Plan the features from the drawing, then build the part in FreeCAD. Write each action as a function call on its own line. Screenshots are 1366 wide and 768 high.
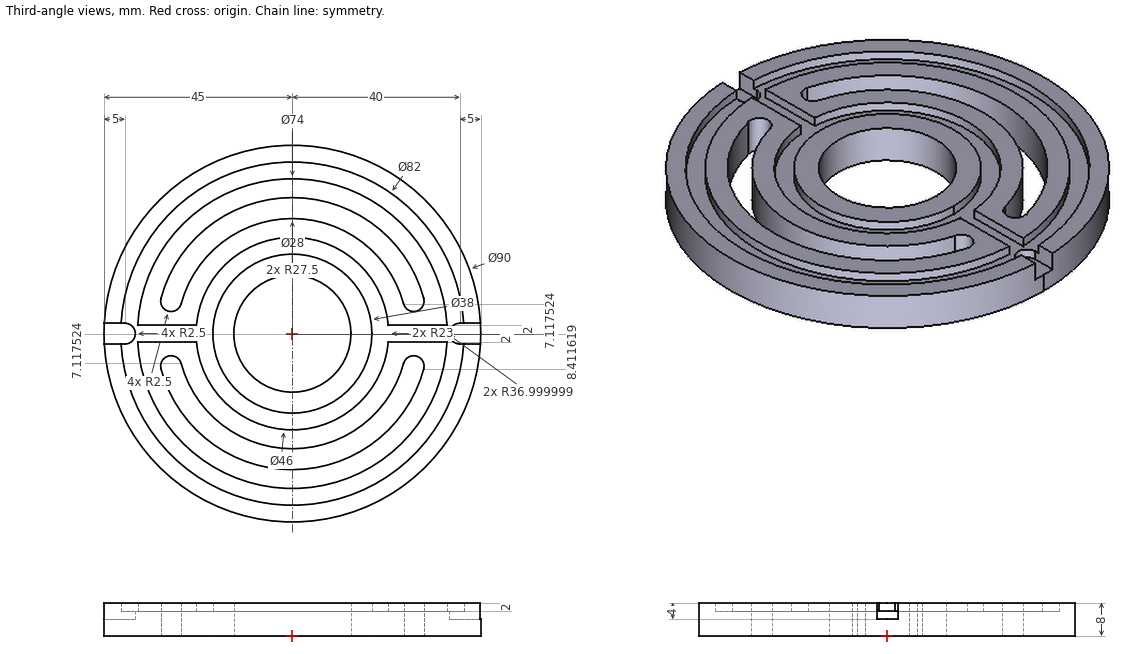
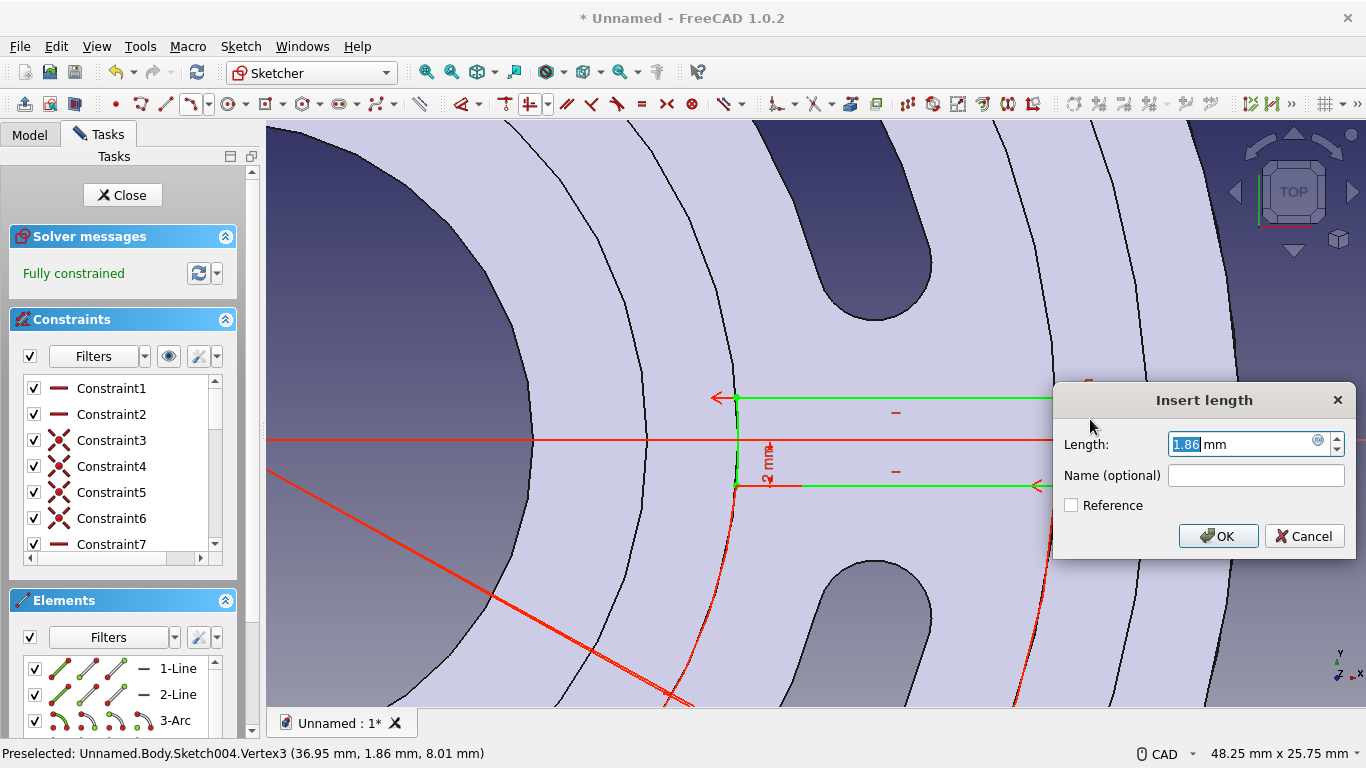
text(2)
key(Return)
key(Escape)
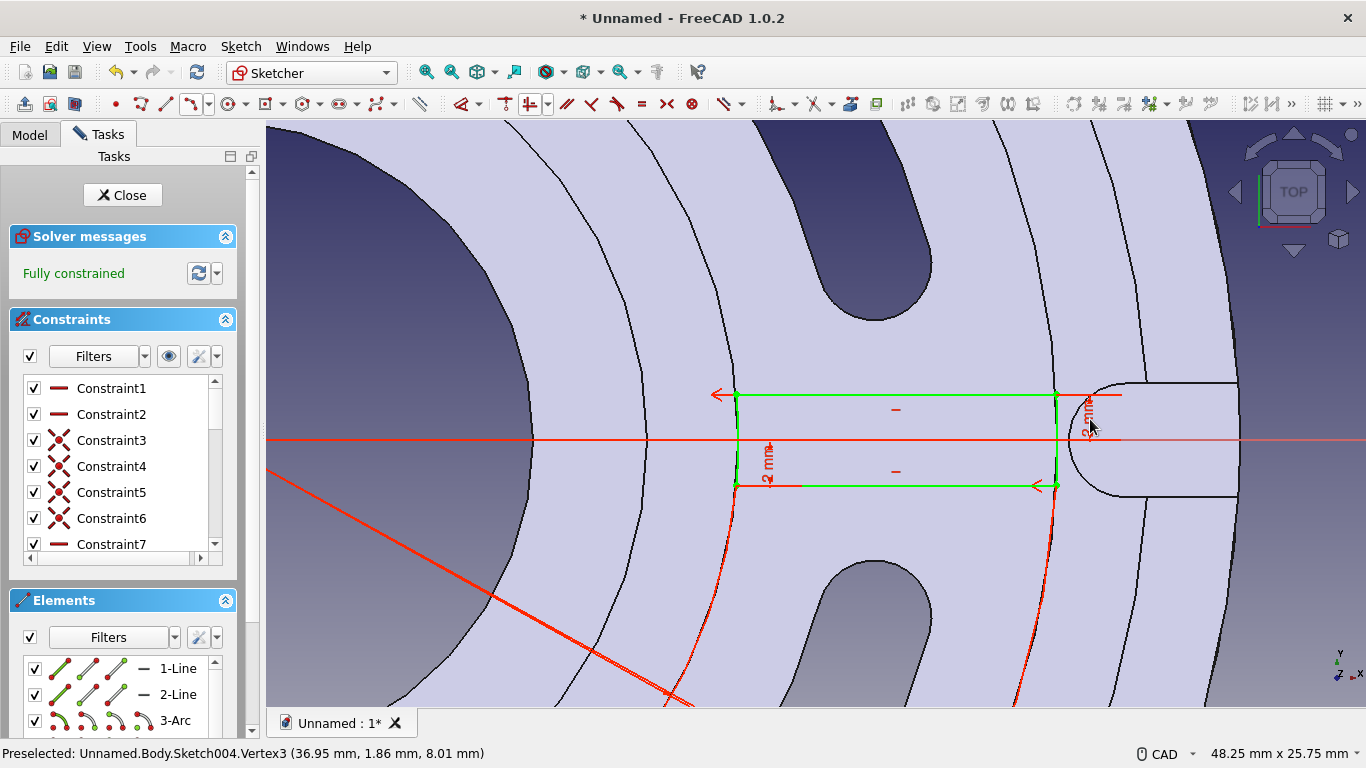
click(123, 195)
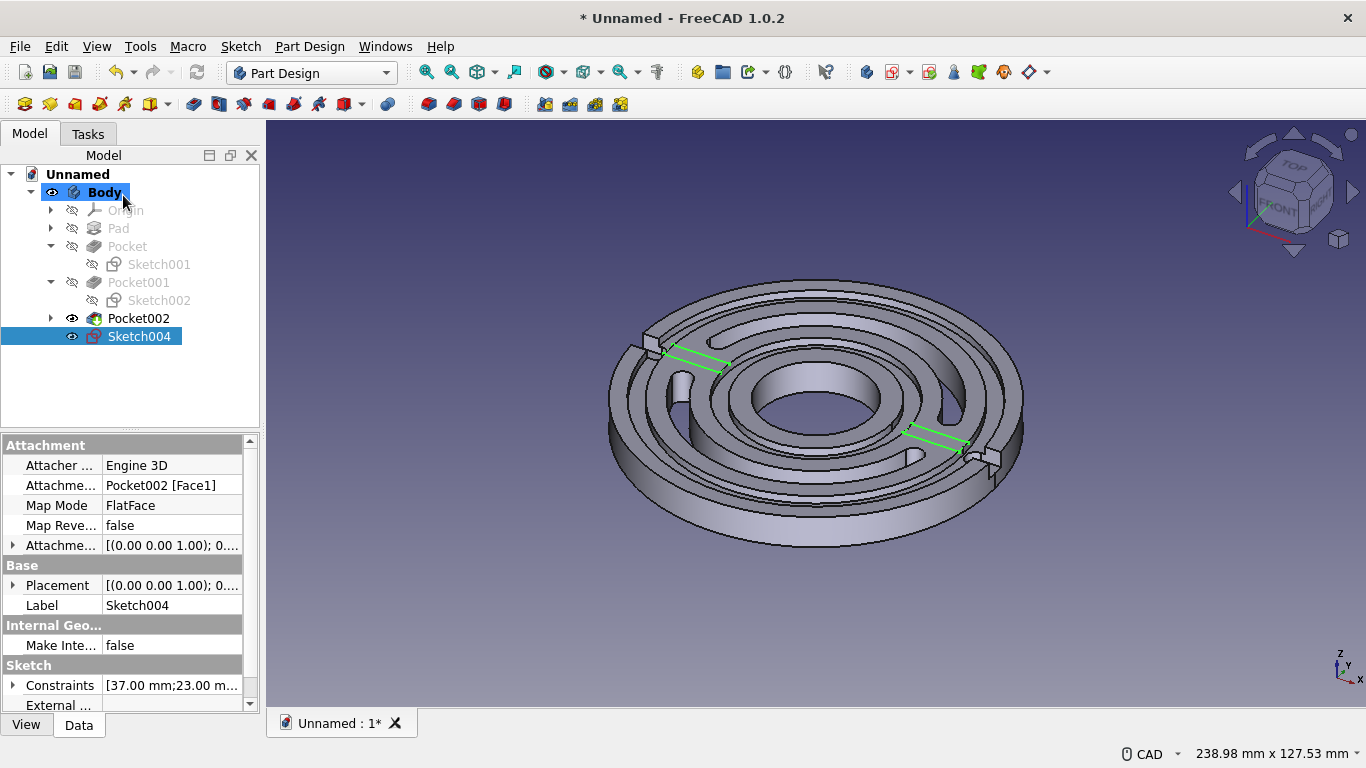
click(194, 104)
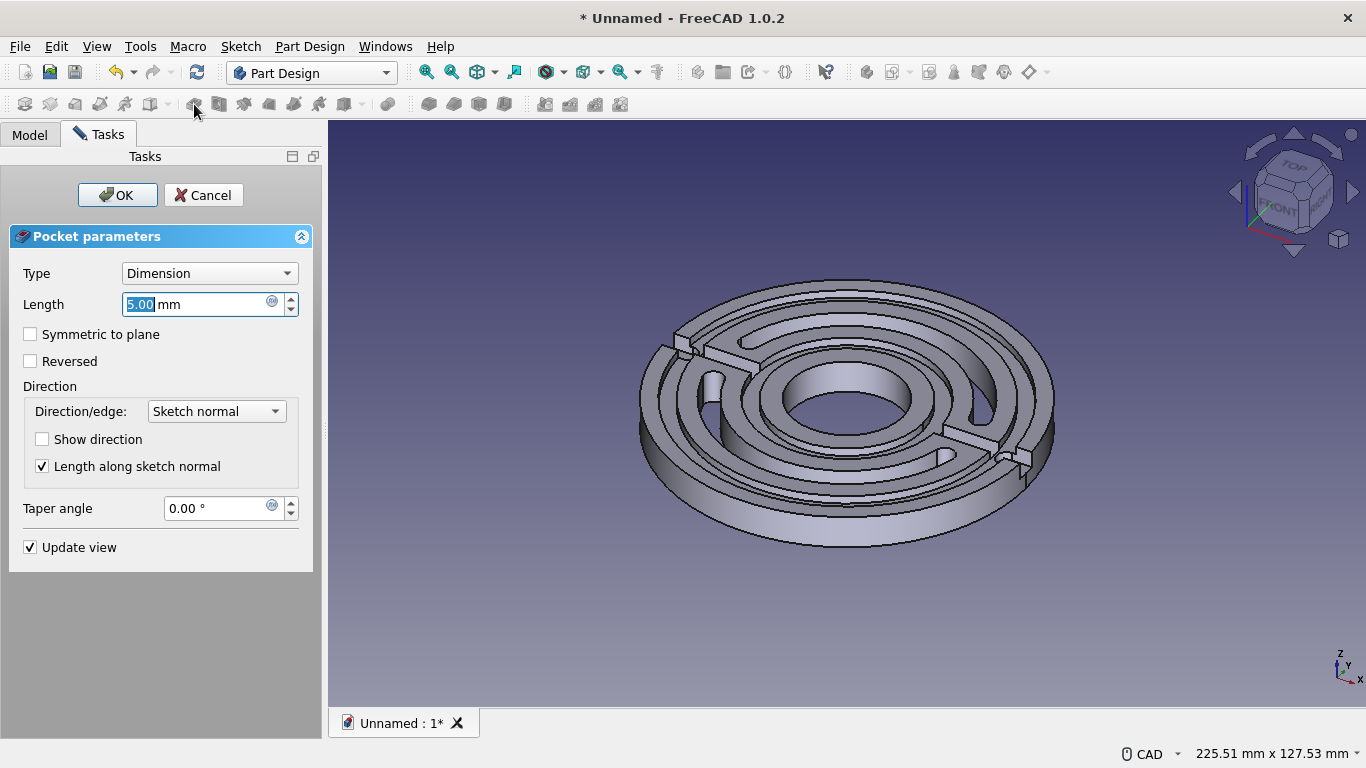
text(2)
key(Tab)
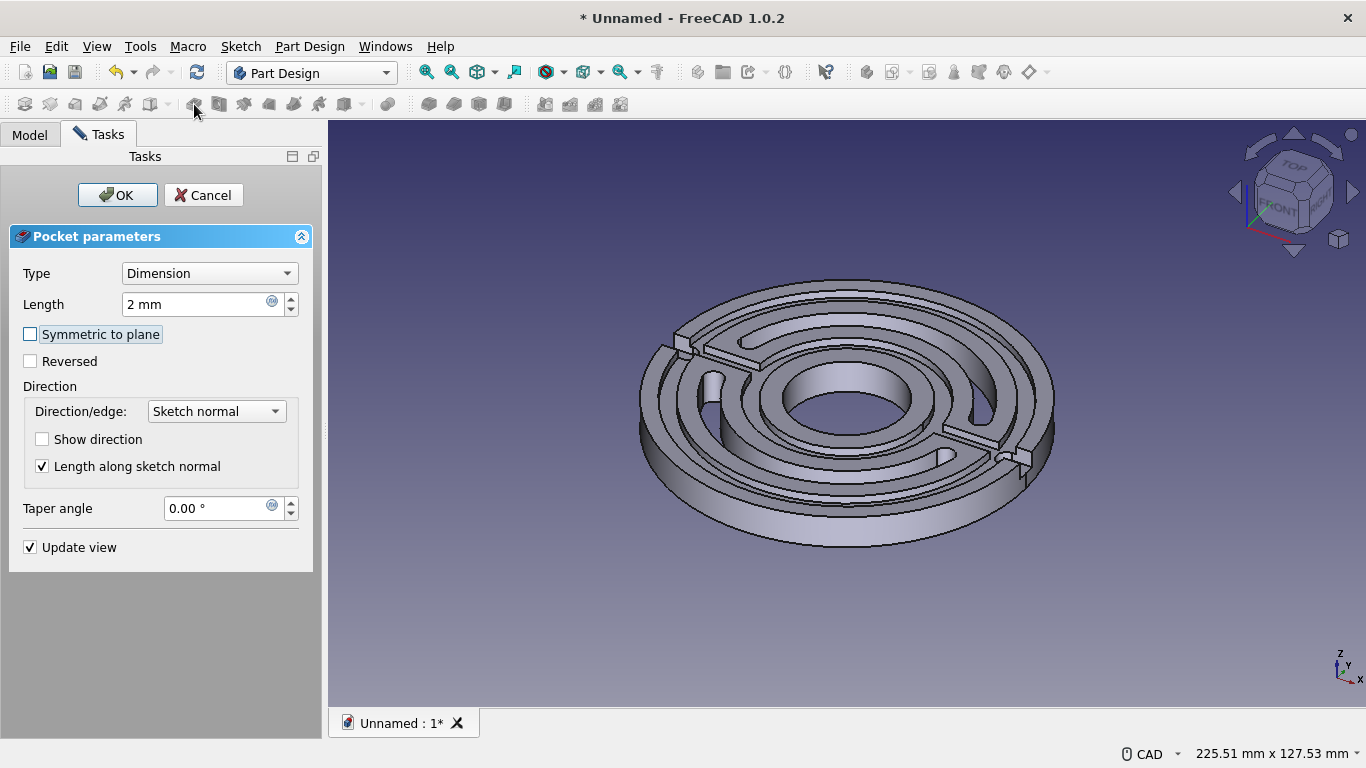
click(118, 195)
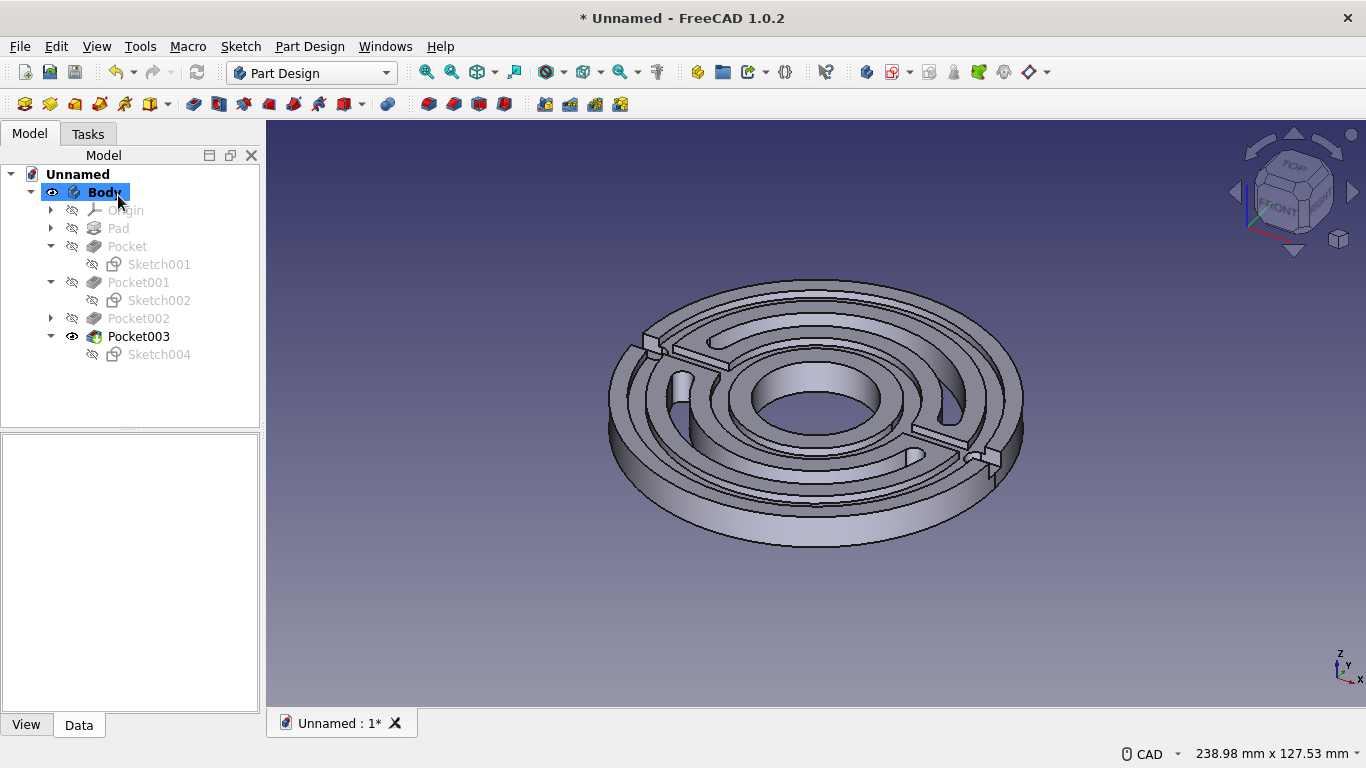
key(0)